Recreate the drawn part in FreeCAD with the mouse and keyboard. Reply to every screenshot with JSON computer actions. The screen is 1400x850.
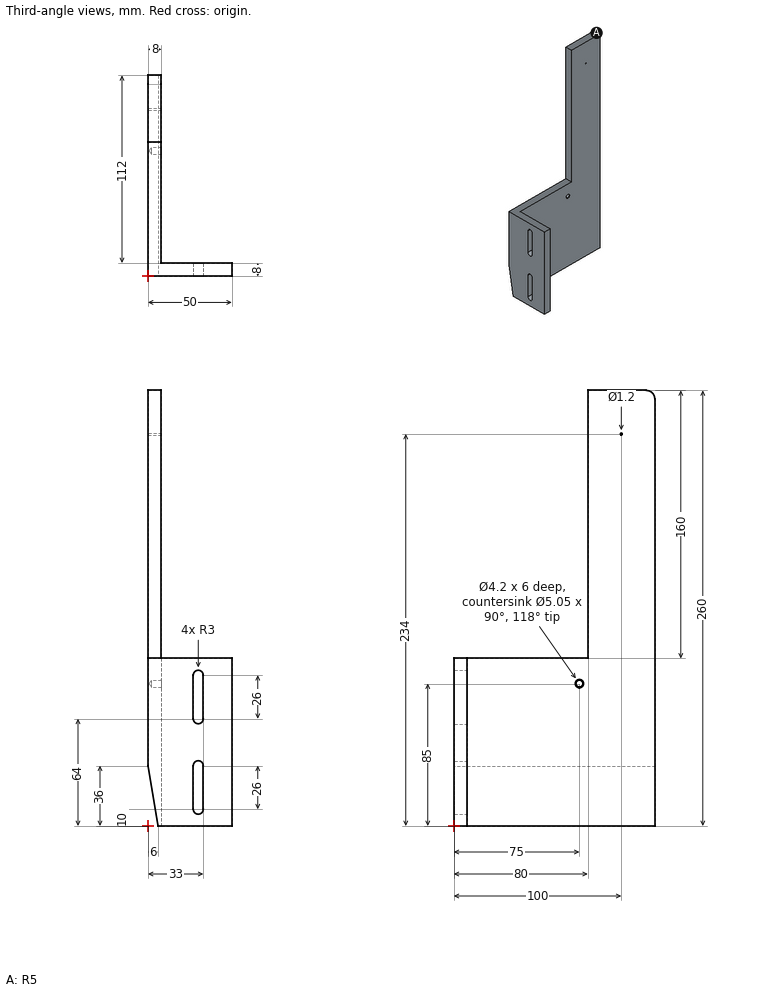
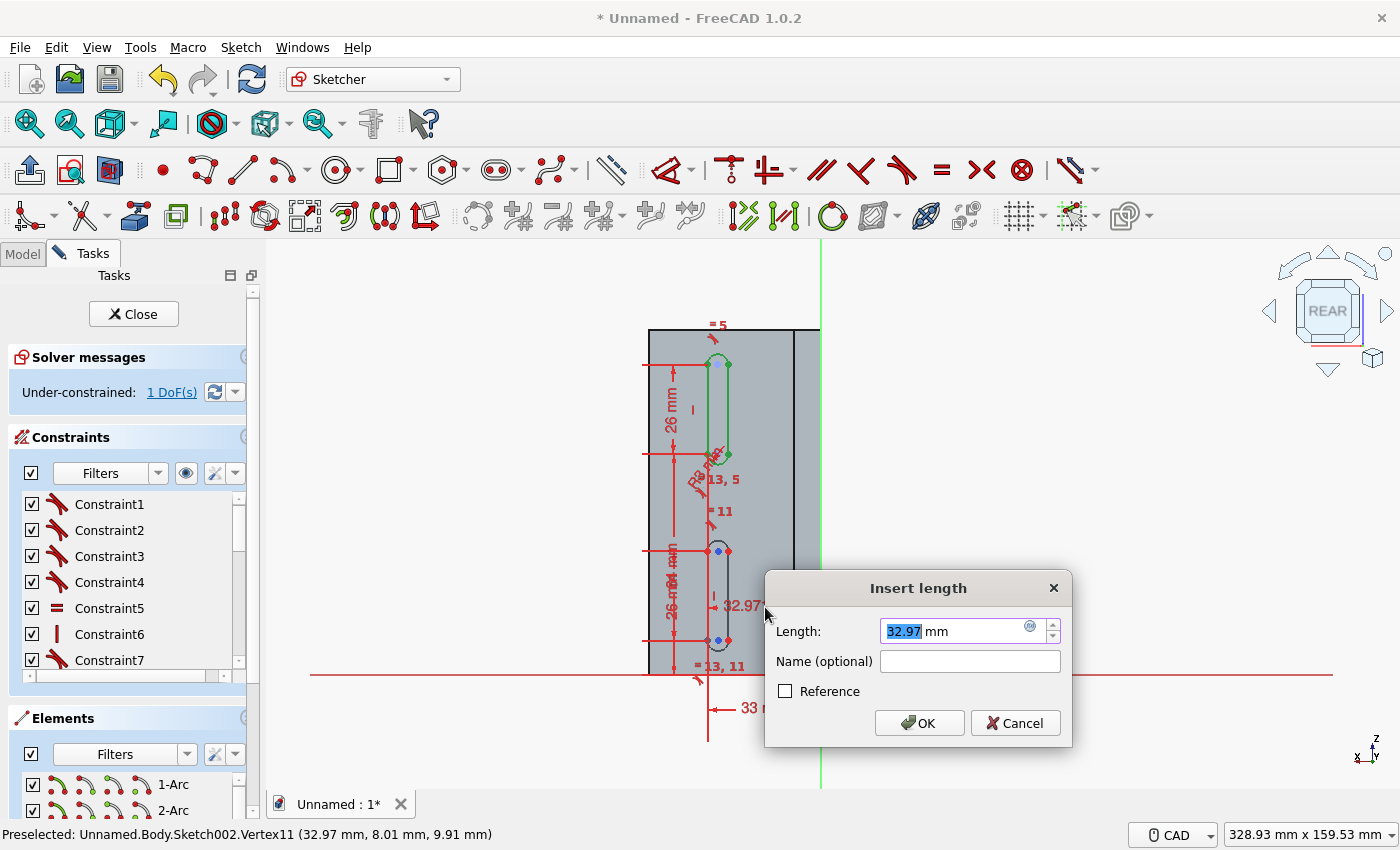
{"action": "type", "text": "33"}
{"action": "key", "text": "Return"}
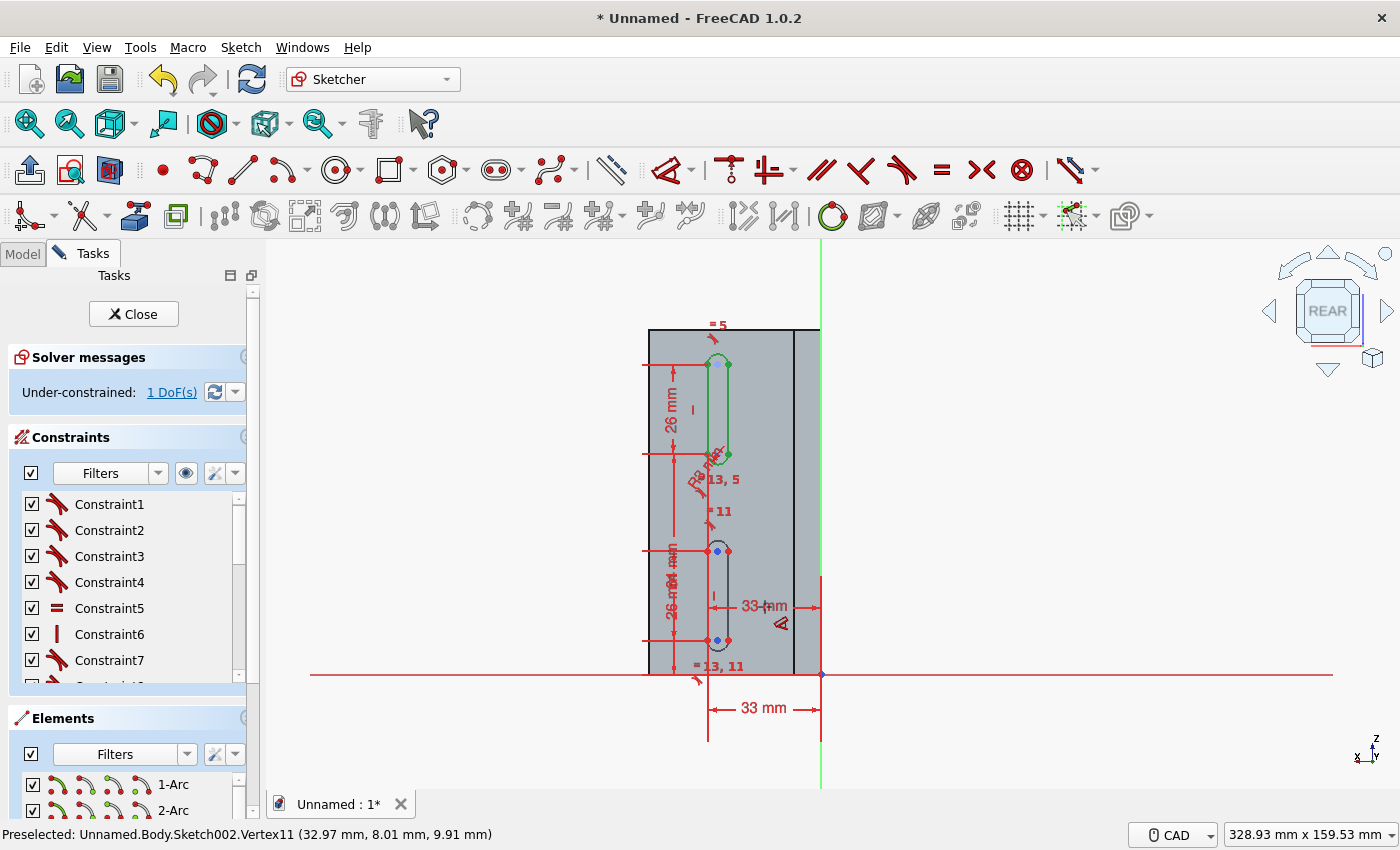
{"action": "left_click", "coordinate": [708, 641]}
{"action": "left_click", "coordinate": [674, 658]}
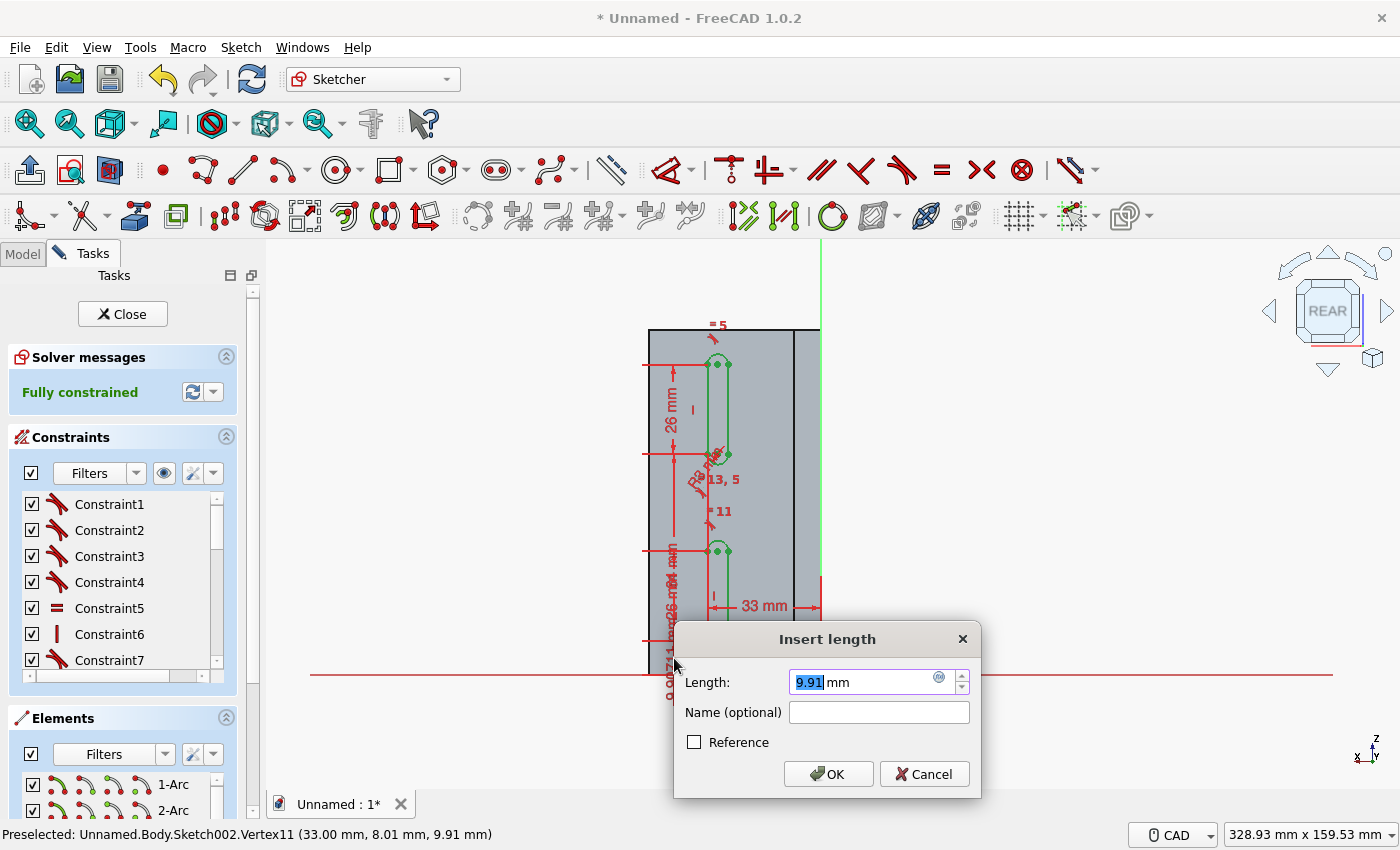
{"action": "type", "text": "10"}
{"action": "key", "text": "Return"}
{"action": "key", "text": "Escape"}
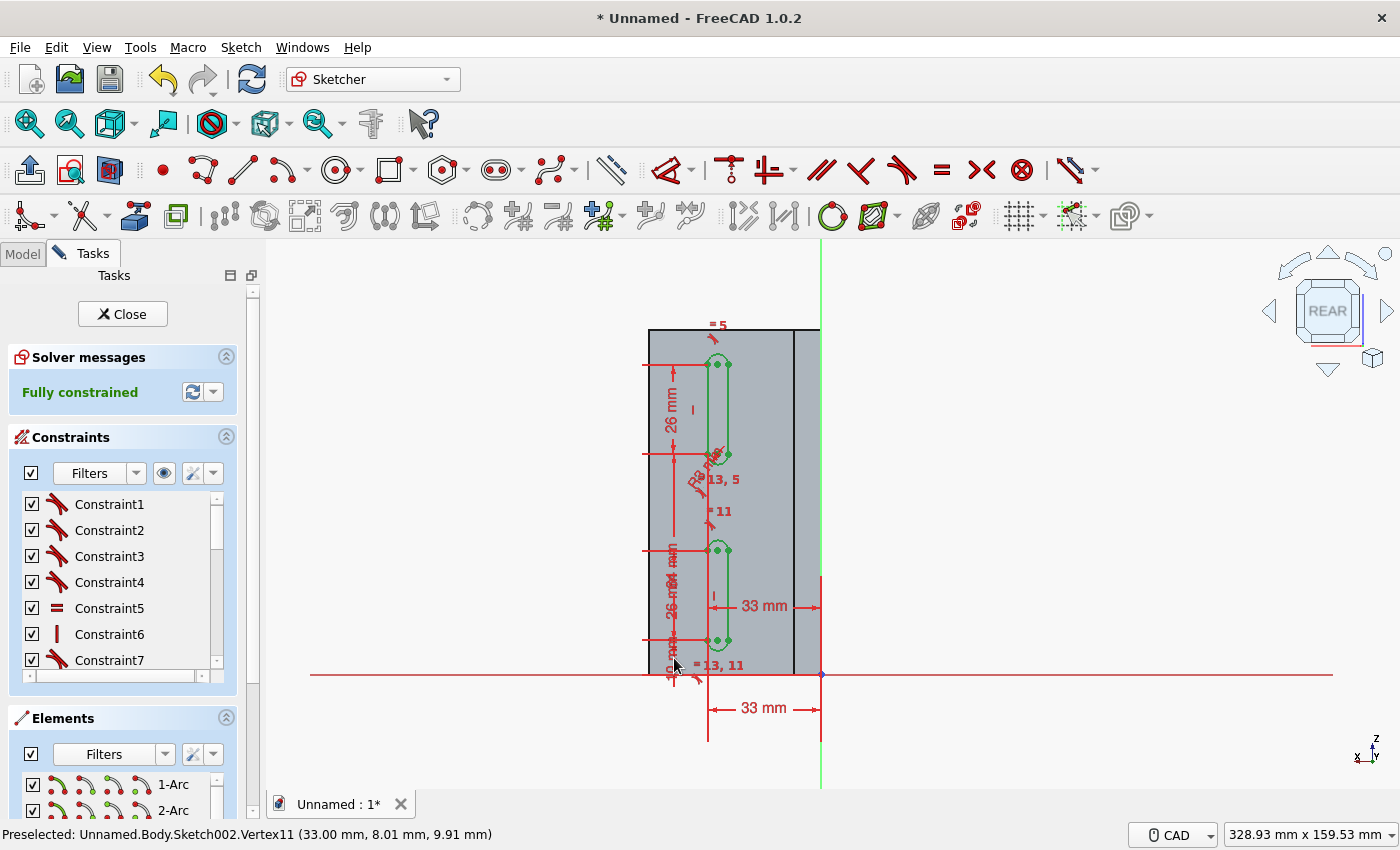
{"action": "left_click", "coordinate": [123, 314]}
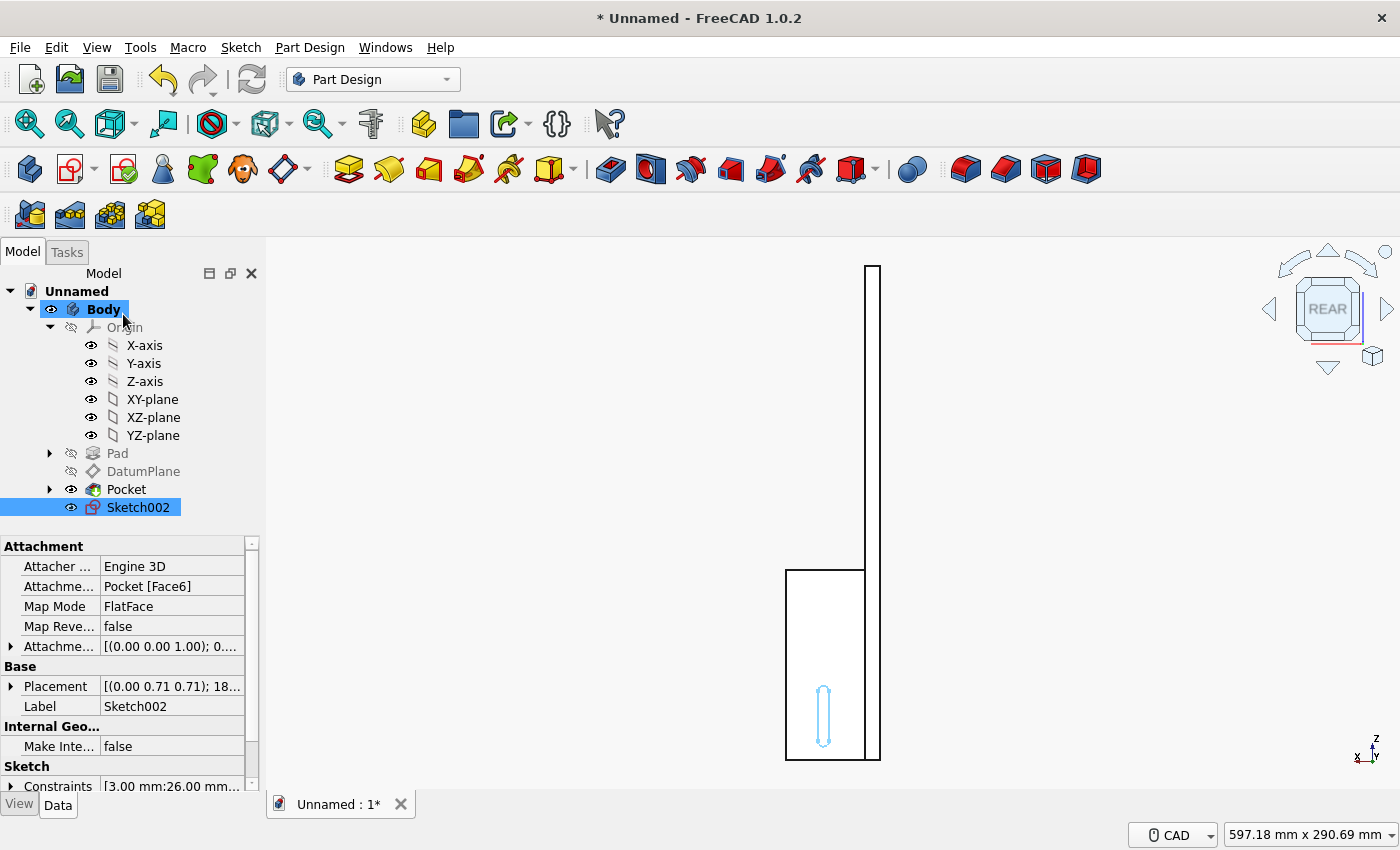
{"action": "left_click", "coordinate": [612, 170]}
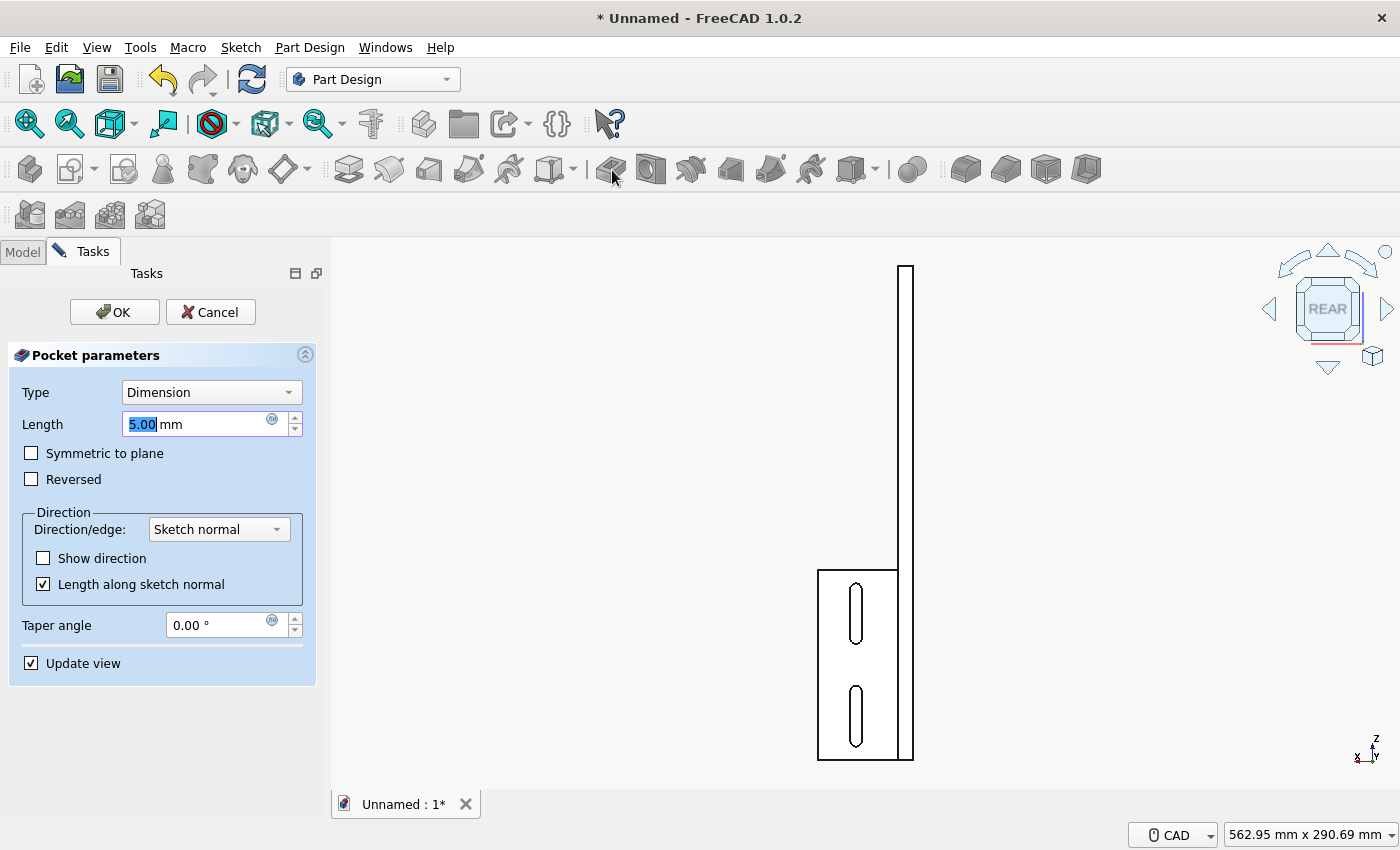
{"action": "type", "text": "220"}
{"action": "key", "text": "Tab"}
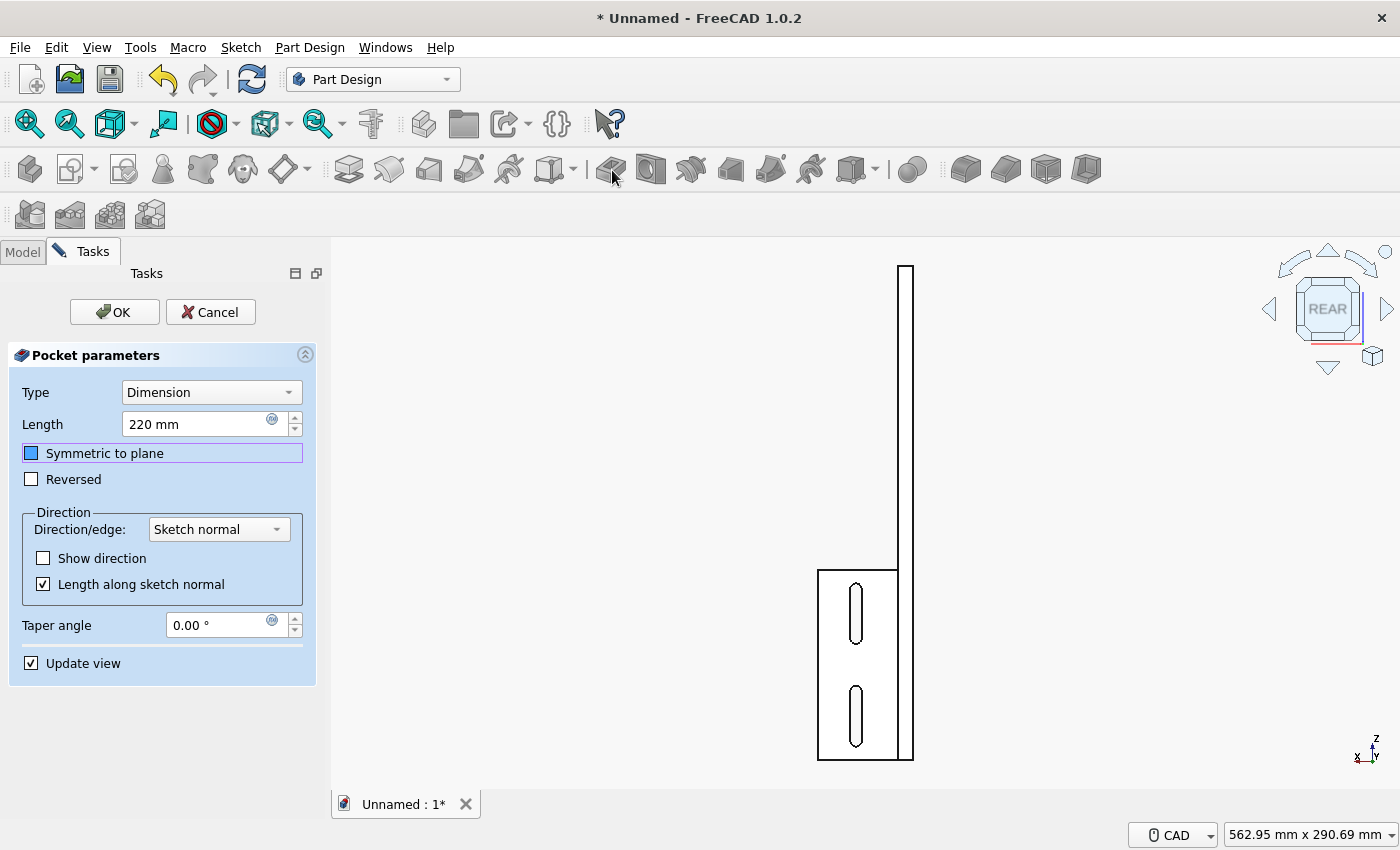
{"action": "left_click", "coordinate": [115, 312]}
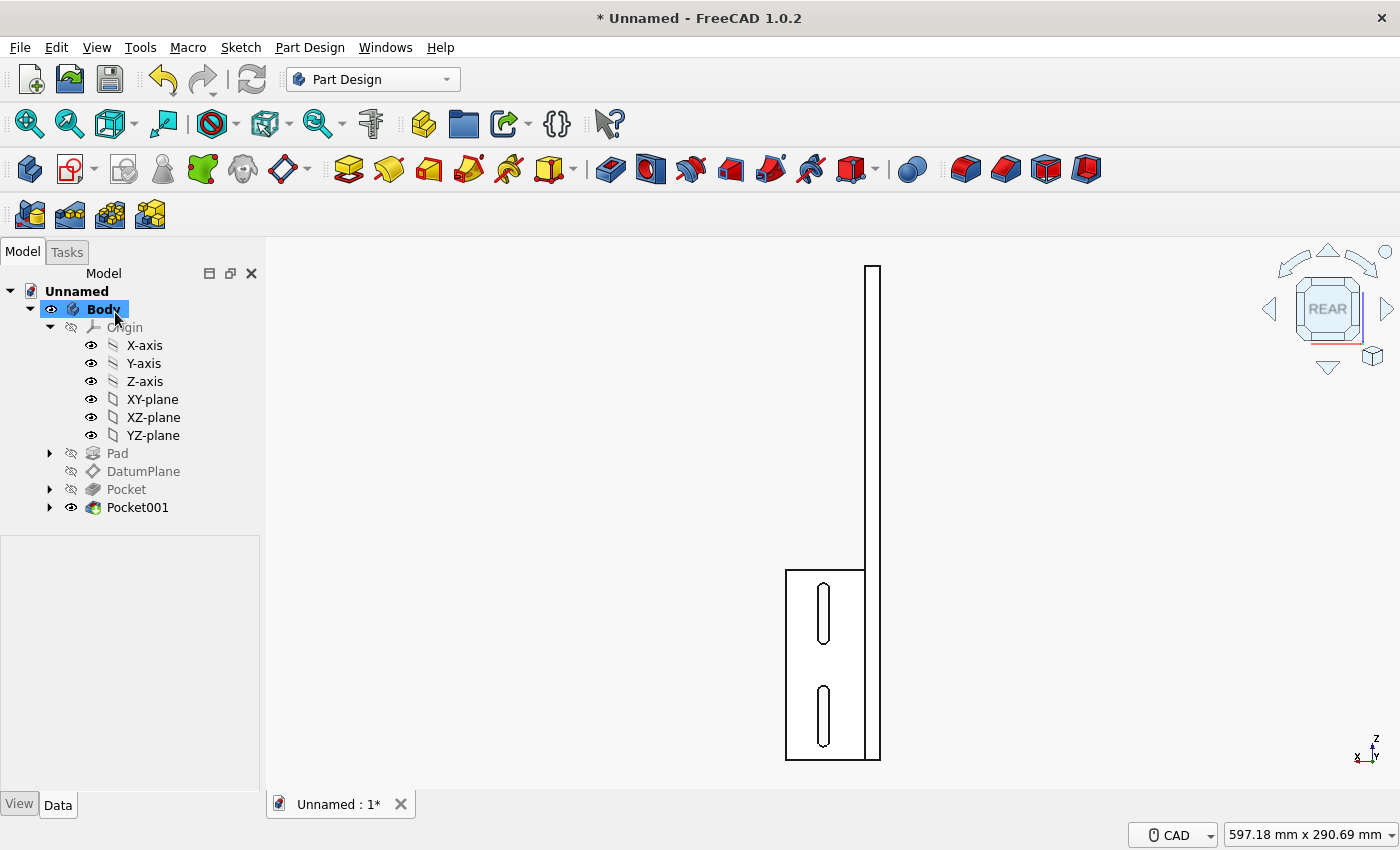
{"action": "left_click", "coordinate": [871, 300]}